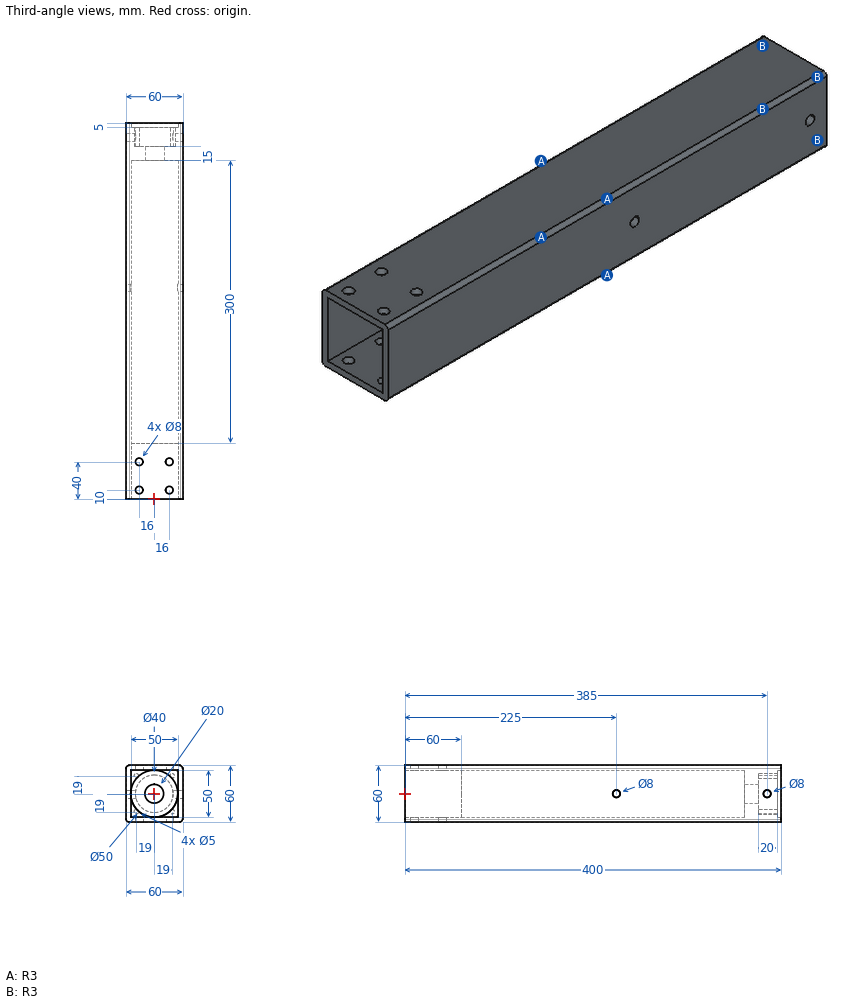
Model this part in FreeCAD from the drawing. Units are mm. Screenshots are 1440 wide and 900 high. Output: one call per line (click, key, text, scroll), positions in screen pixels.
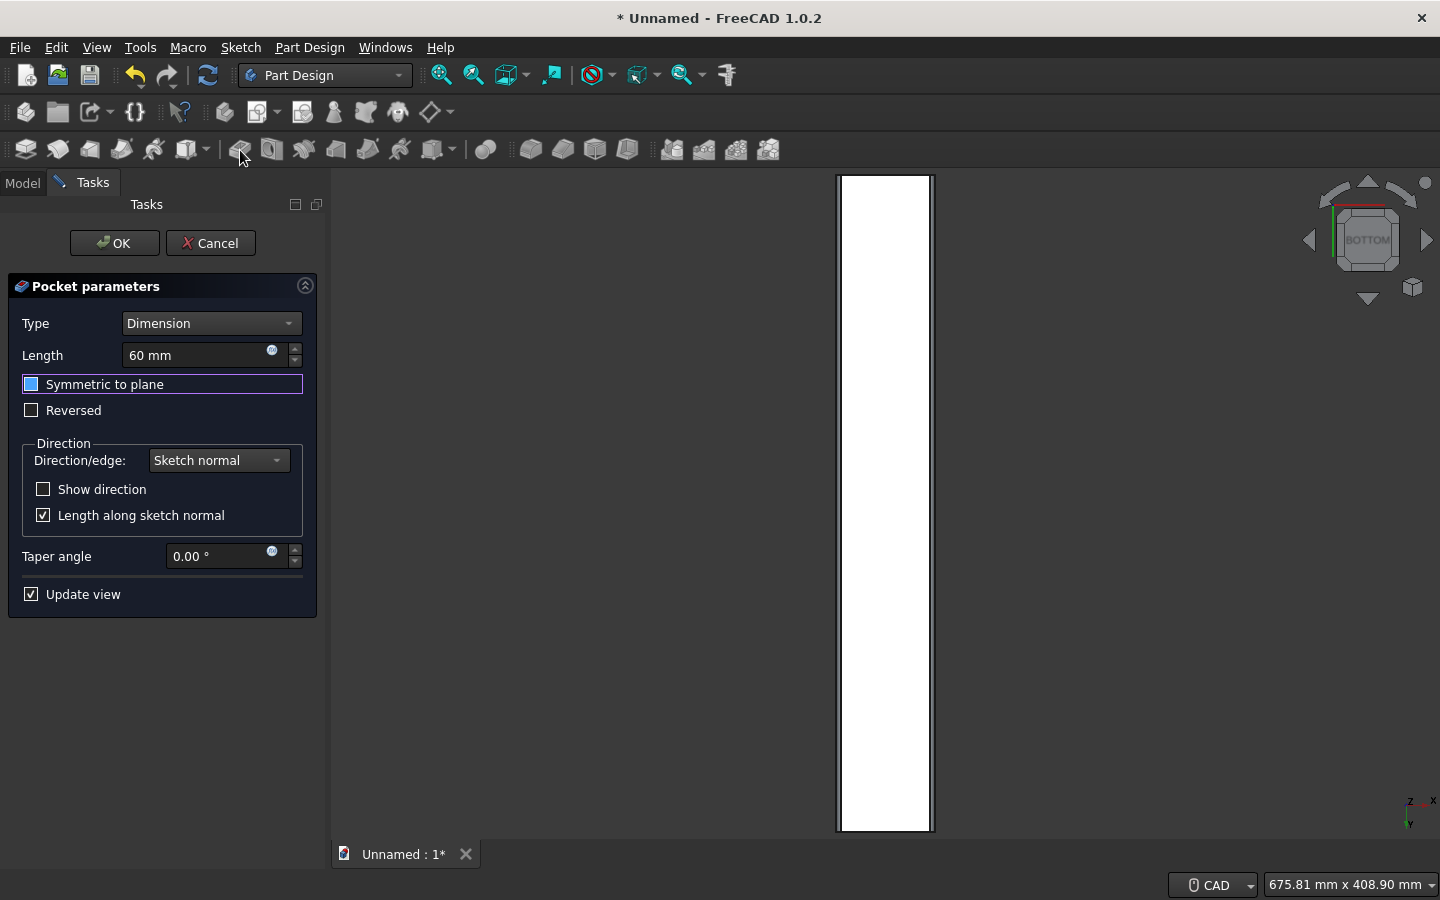
click(30, 384)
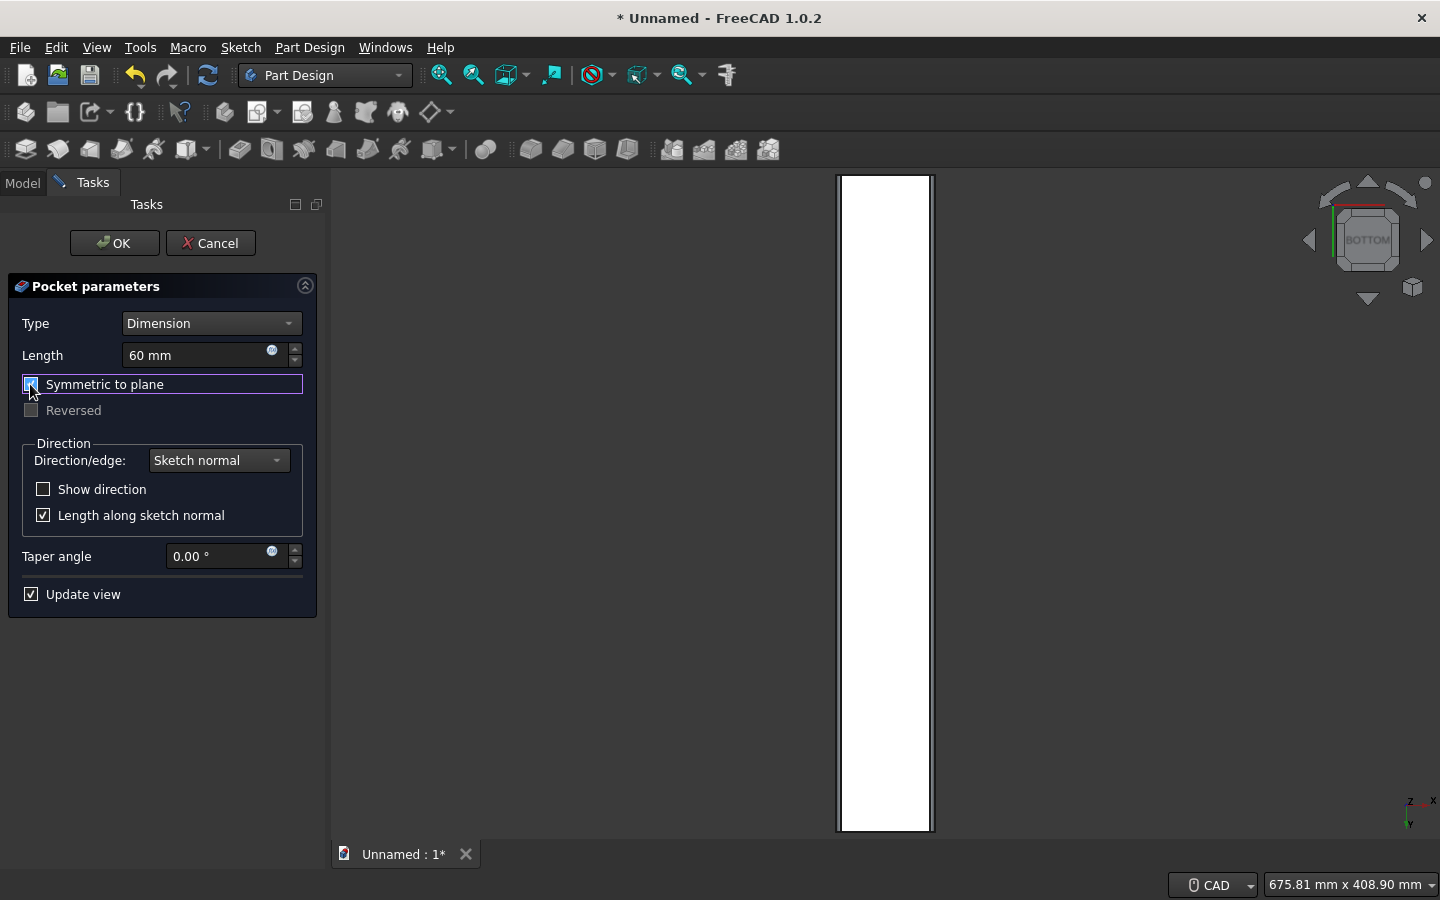
click(115, 243)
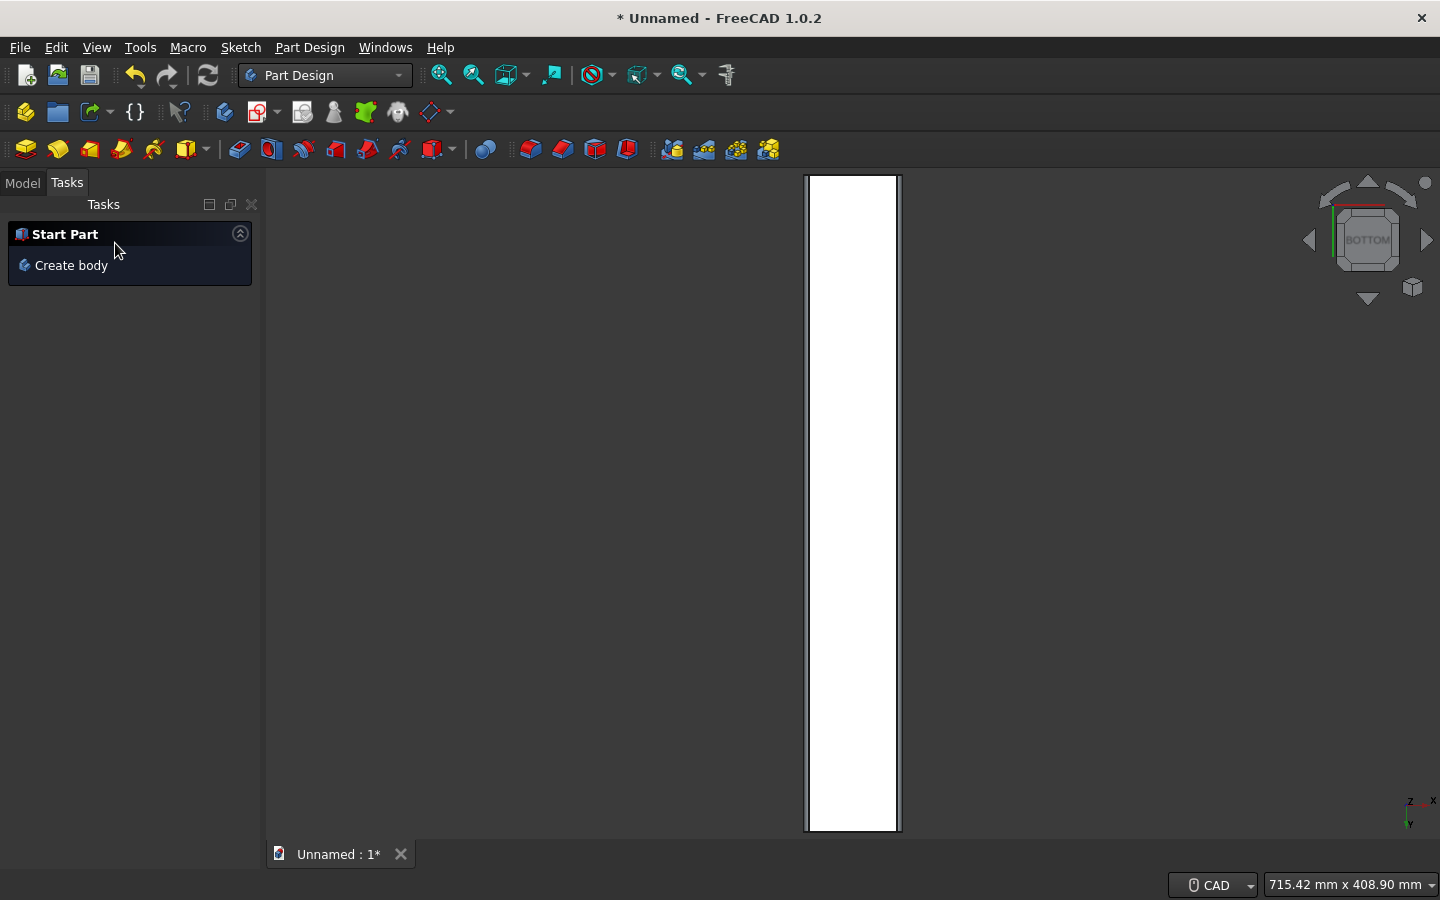
key(0)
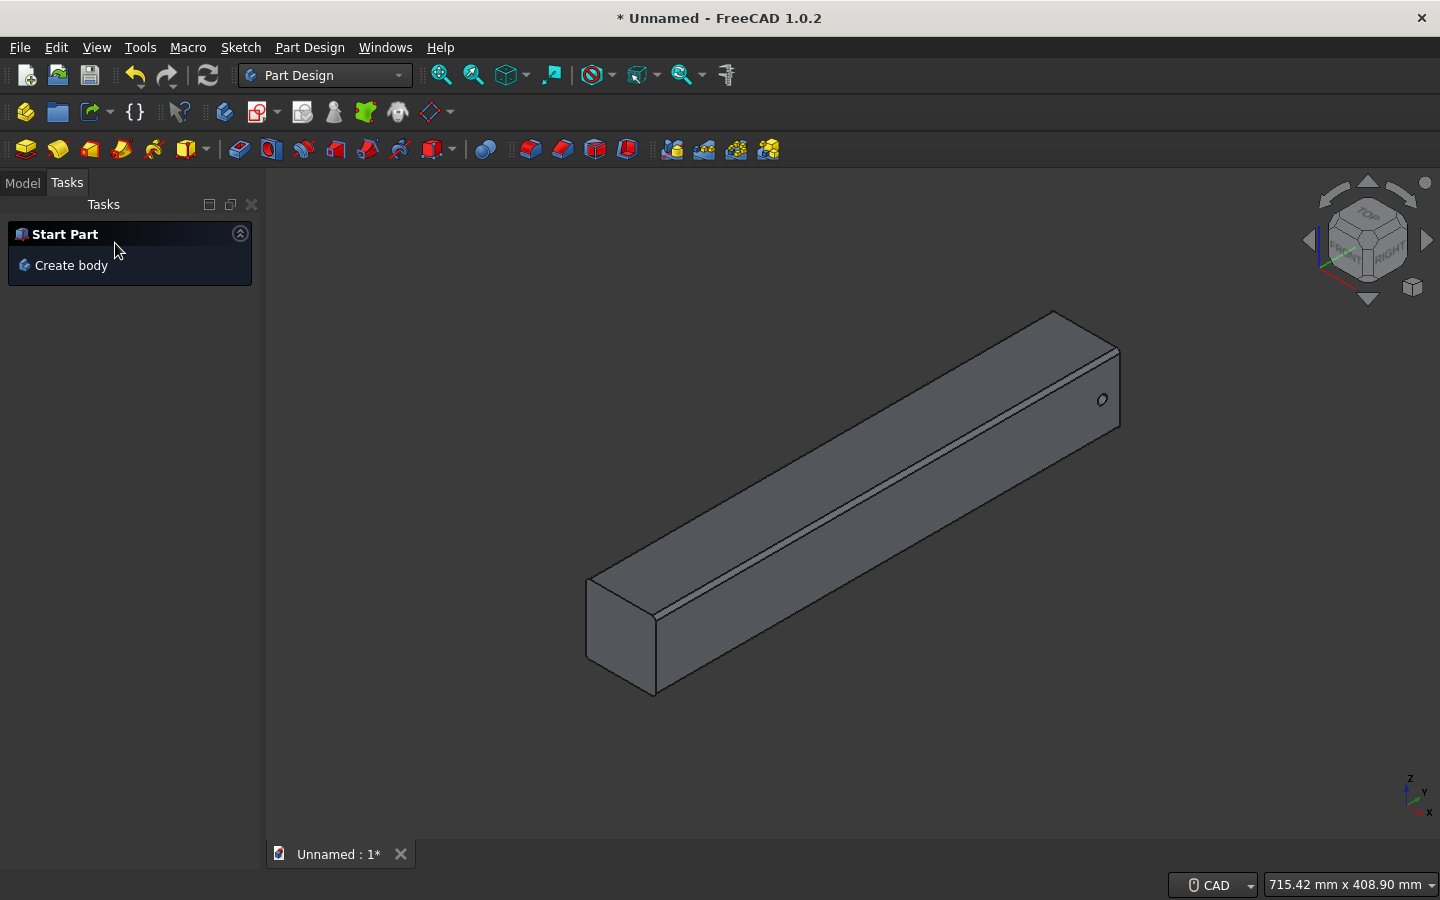
click(621, 636)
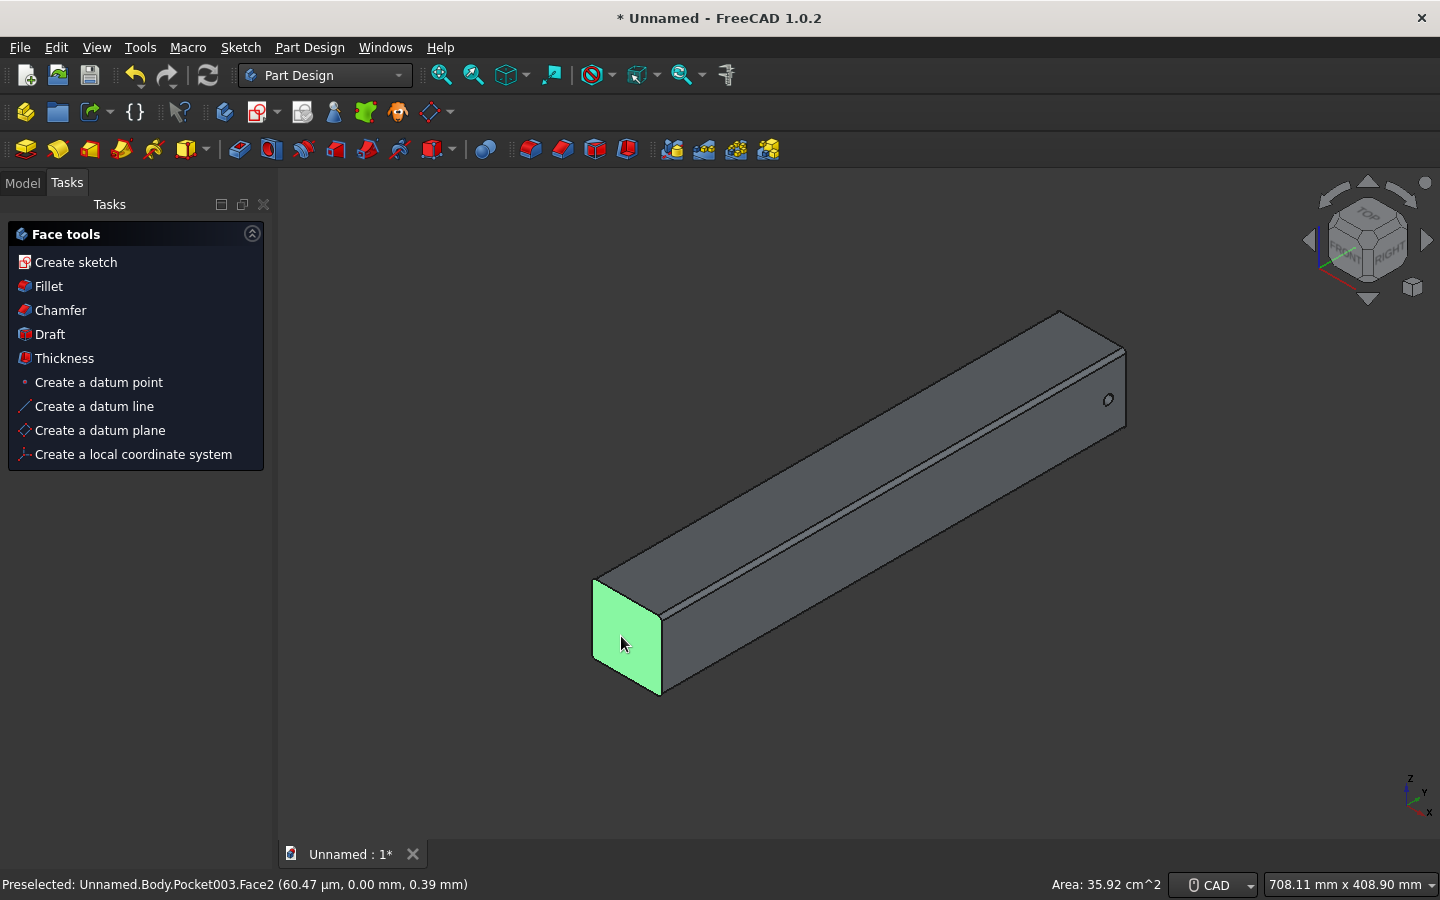
click(258, 112)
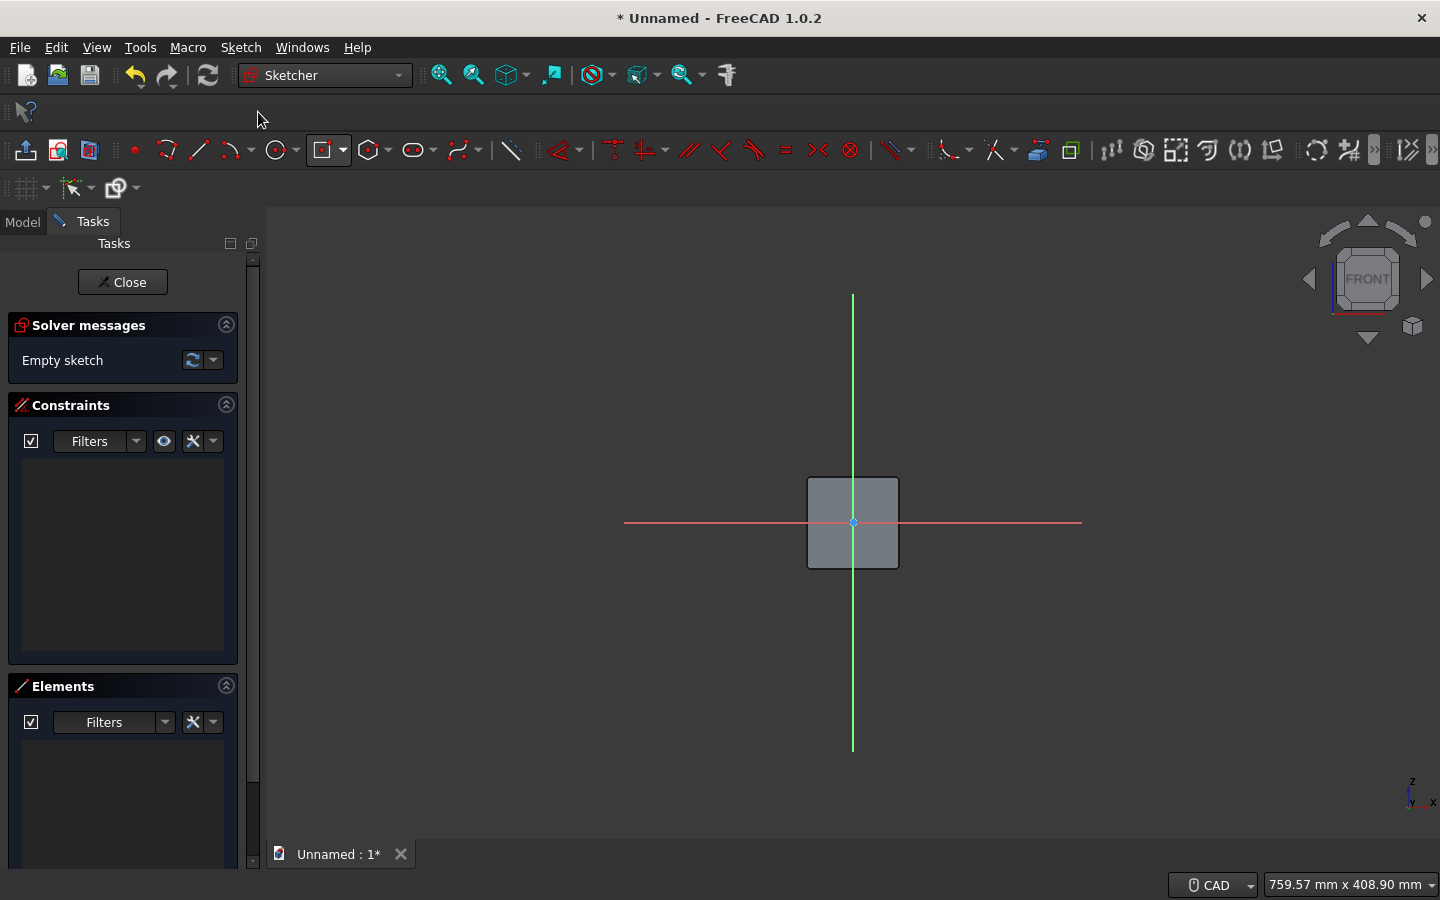
scroll(870, 523, up, 8)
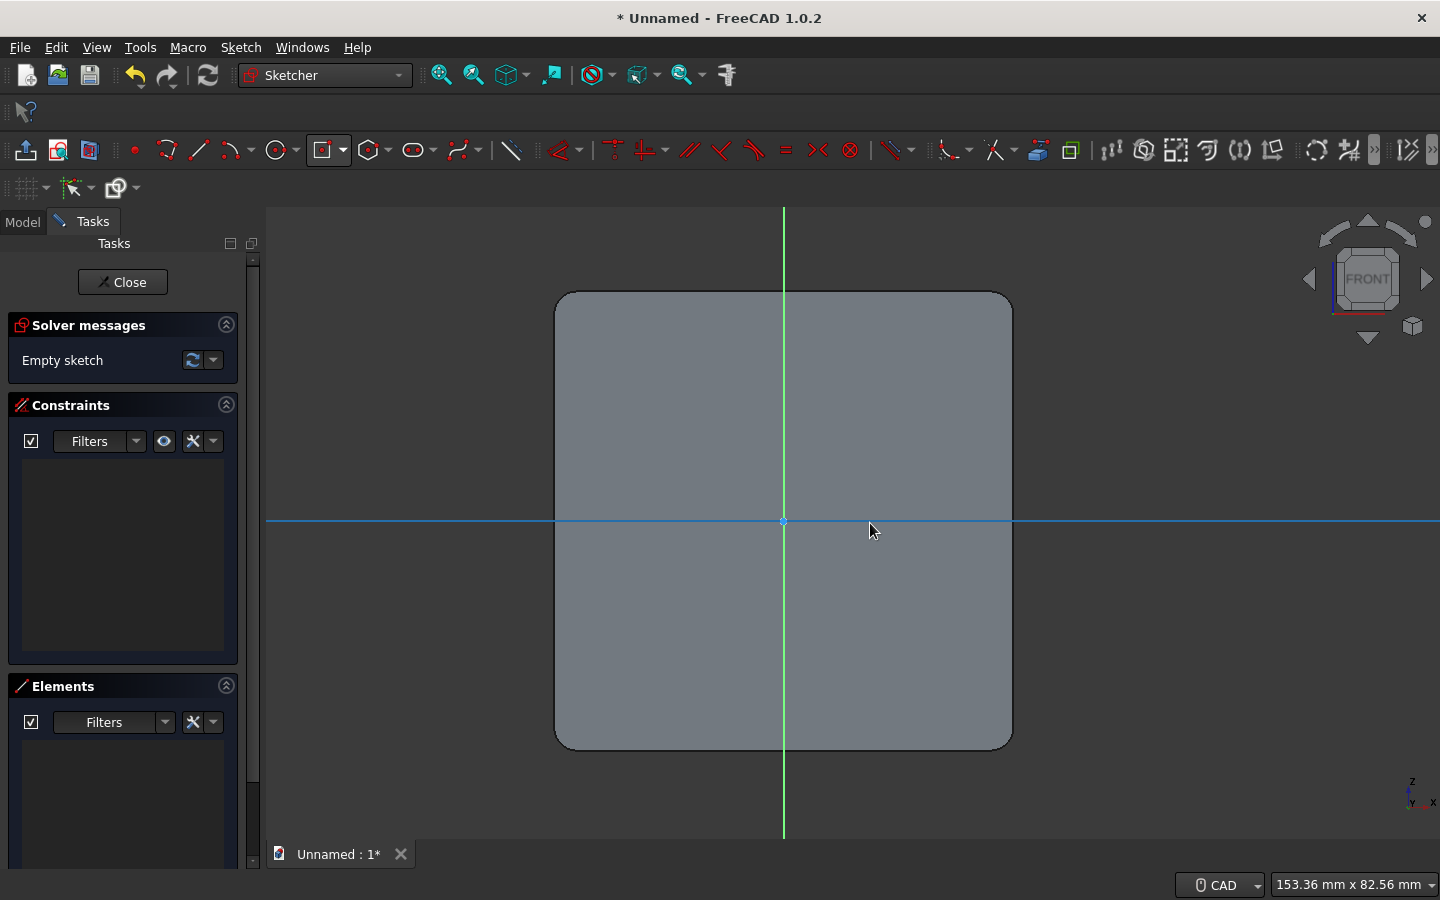
click(322, 150)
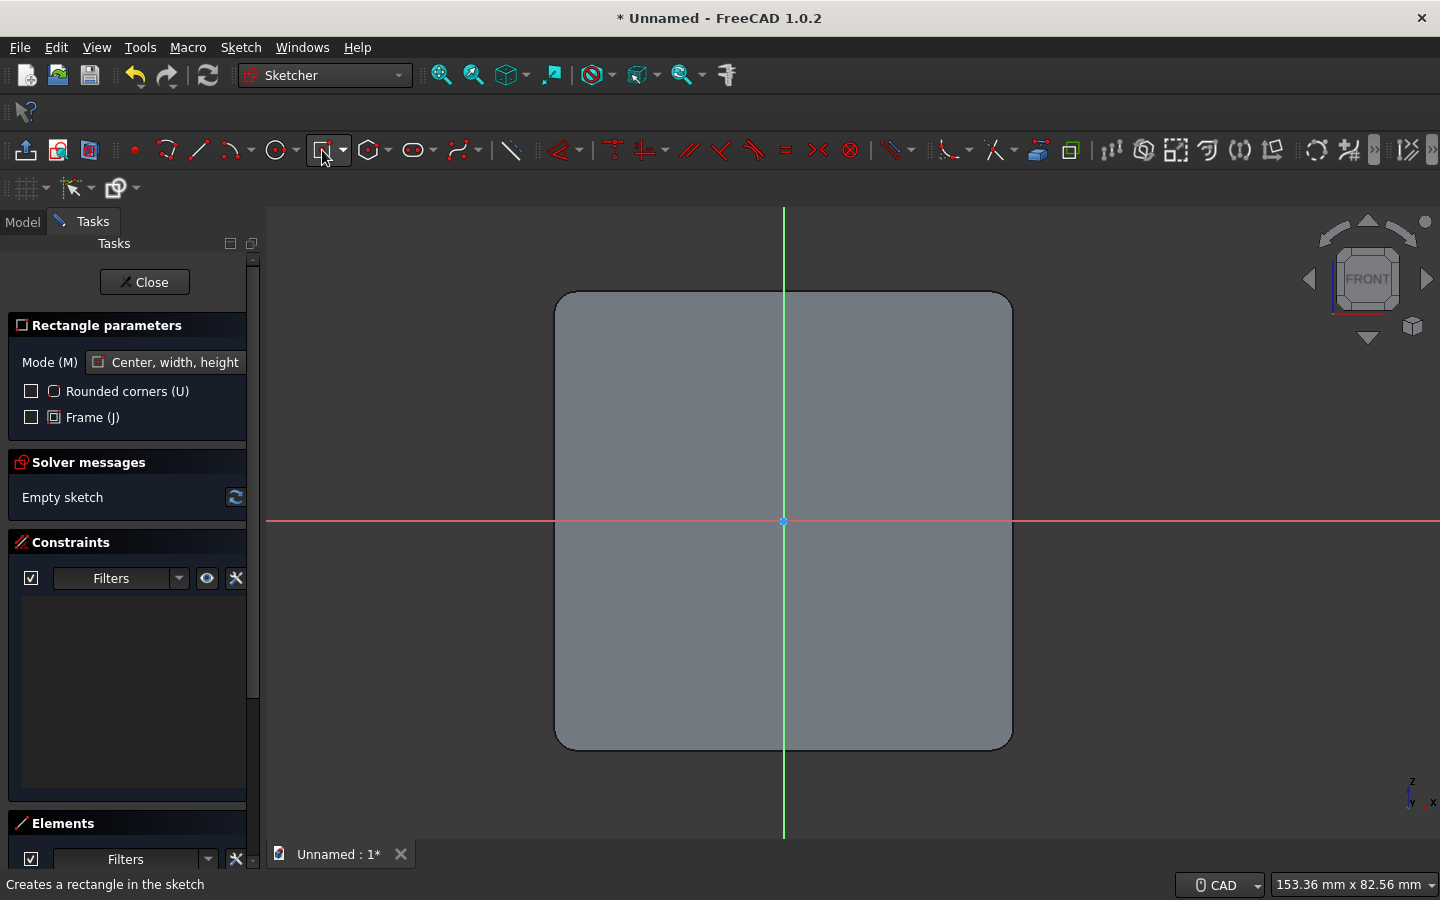
click(784, 521)
move(975, 330)